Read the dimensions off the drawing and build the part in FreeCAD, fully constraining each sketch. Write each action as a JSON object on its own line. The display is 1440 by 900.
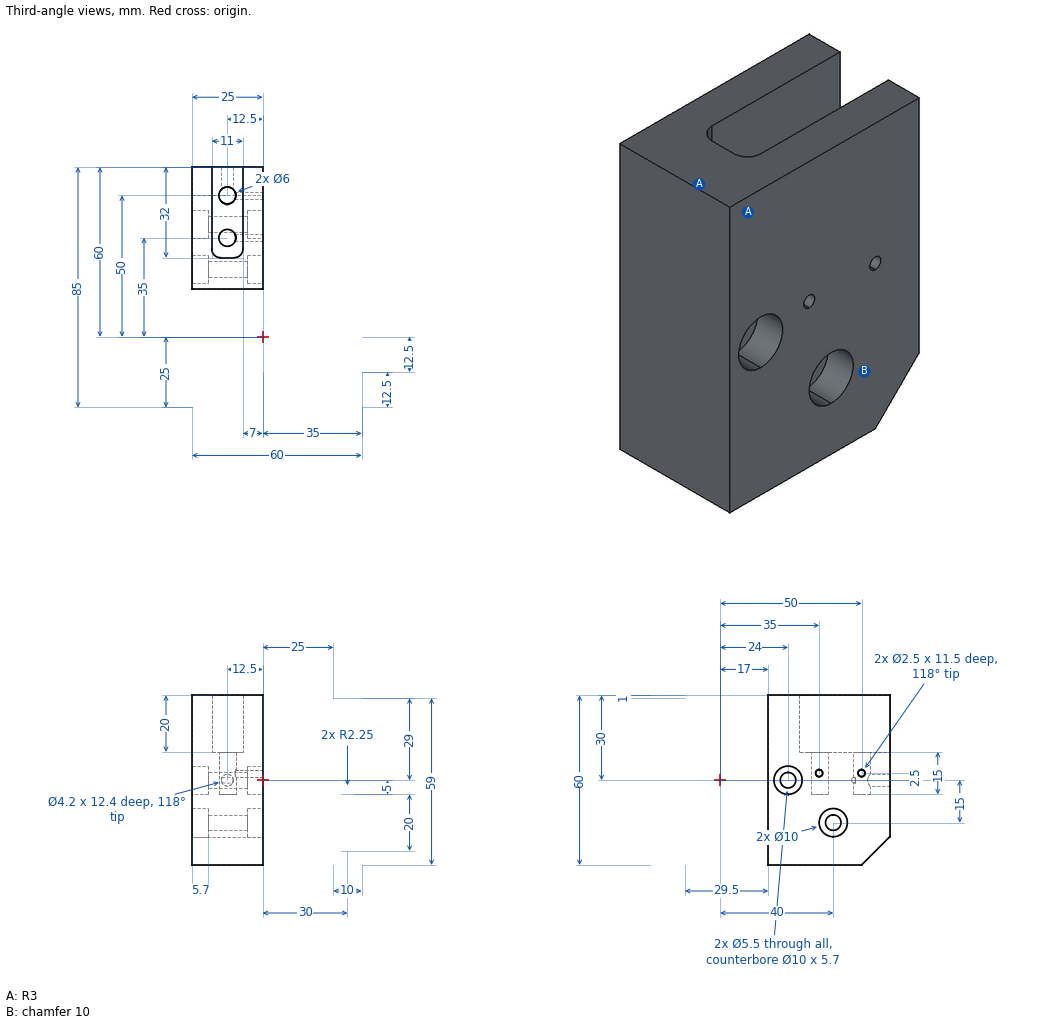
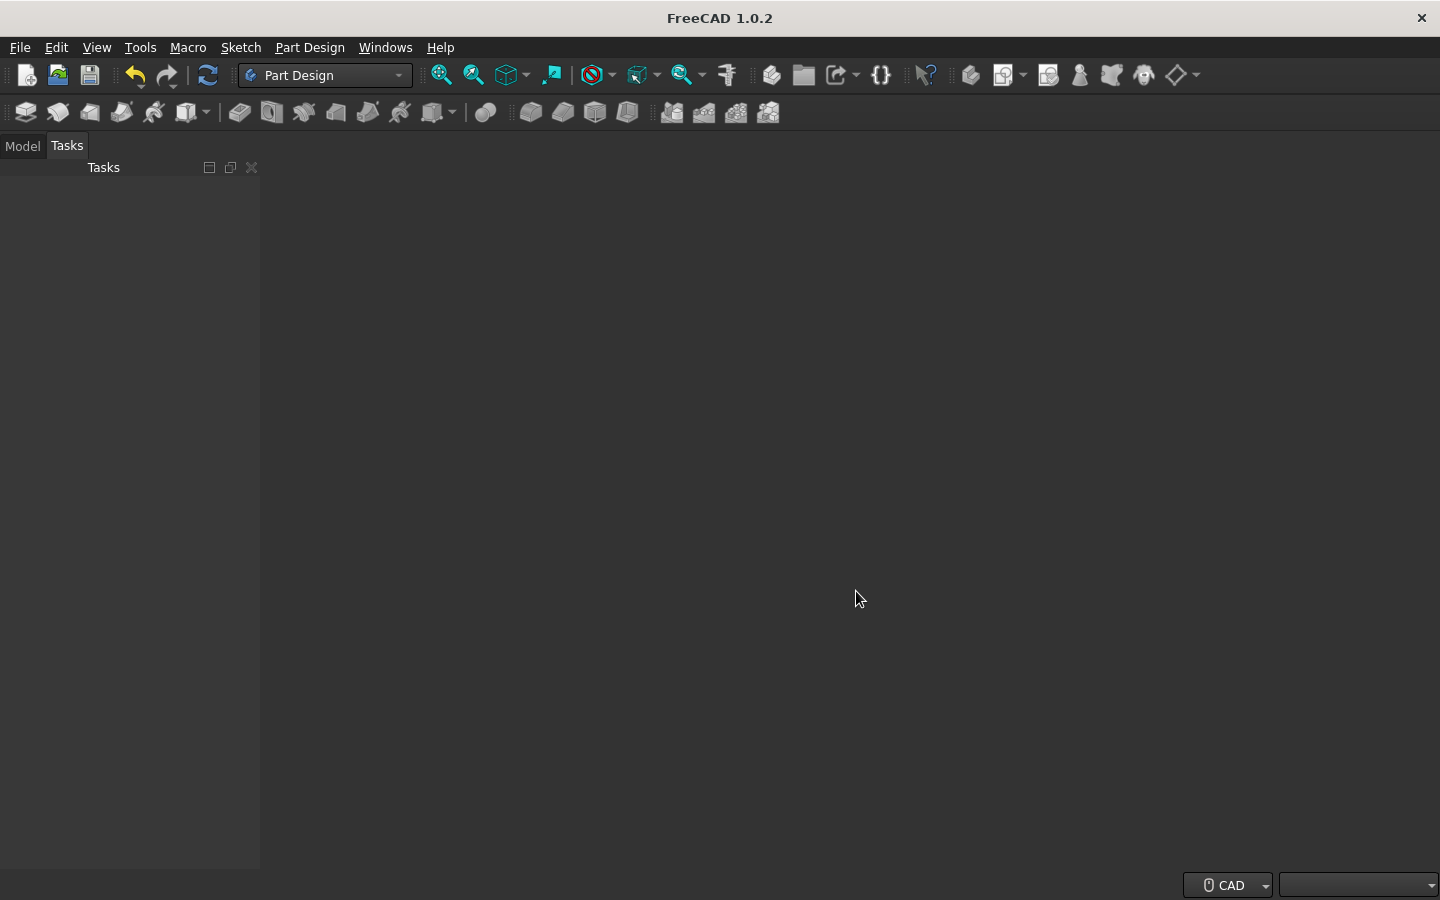
{"action": "left_click", "coordinate": [26, 76]}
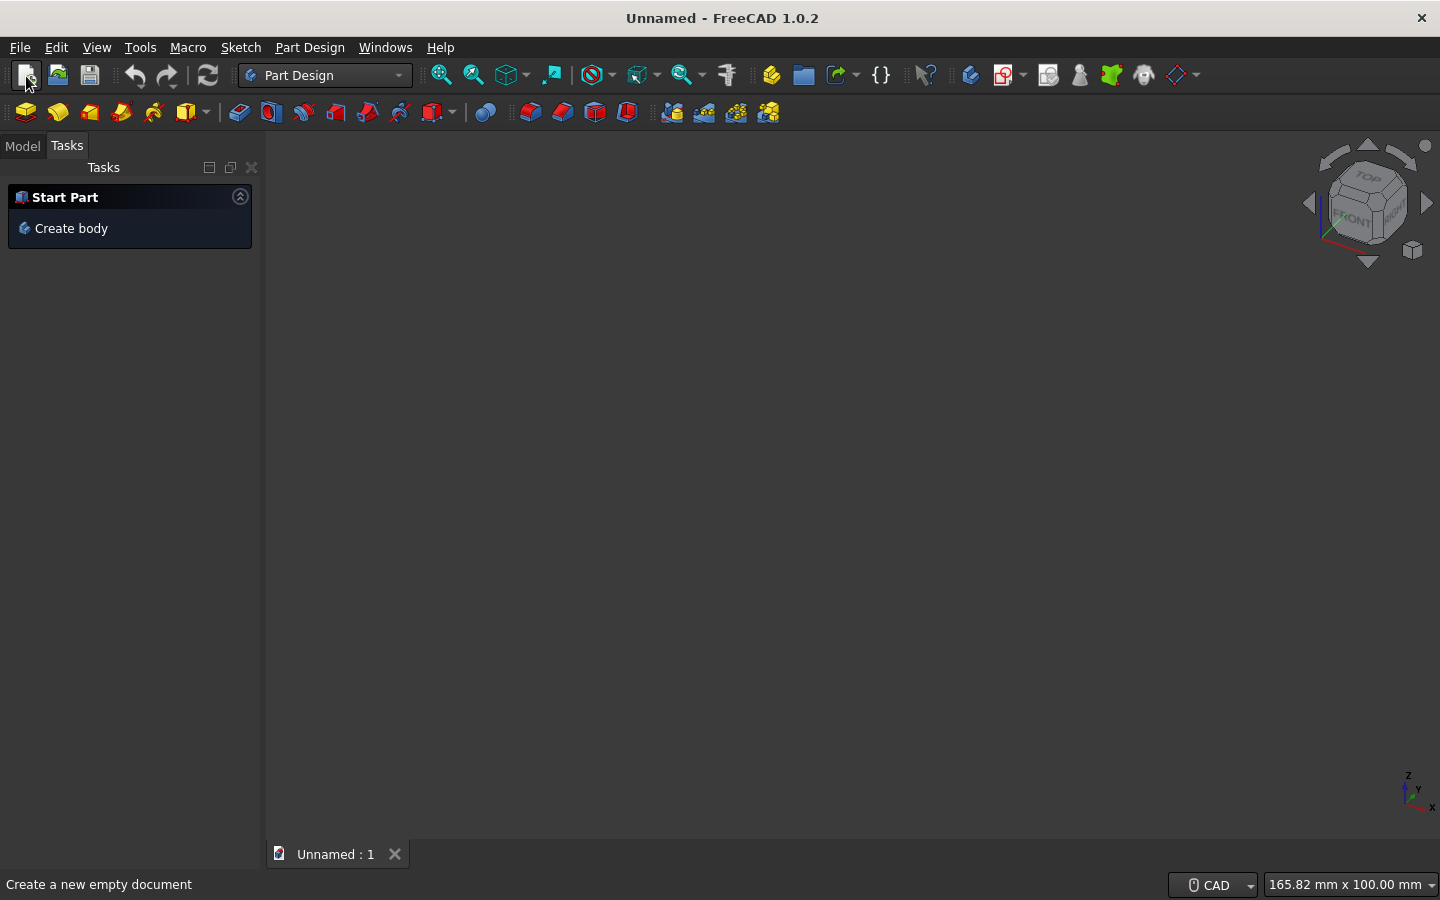
{"action": "left_click", "coordinate": [1004, 76]}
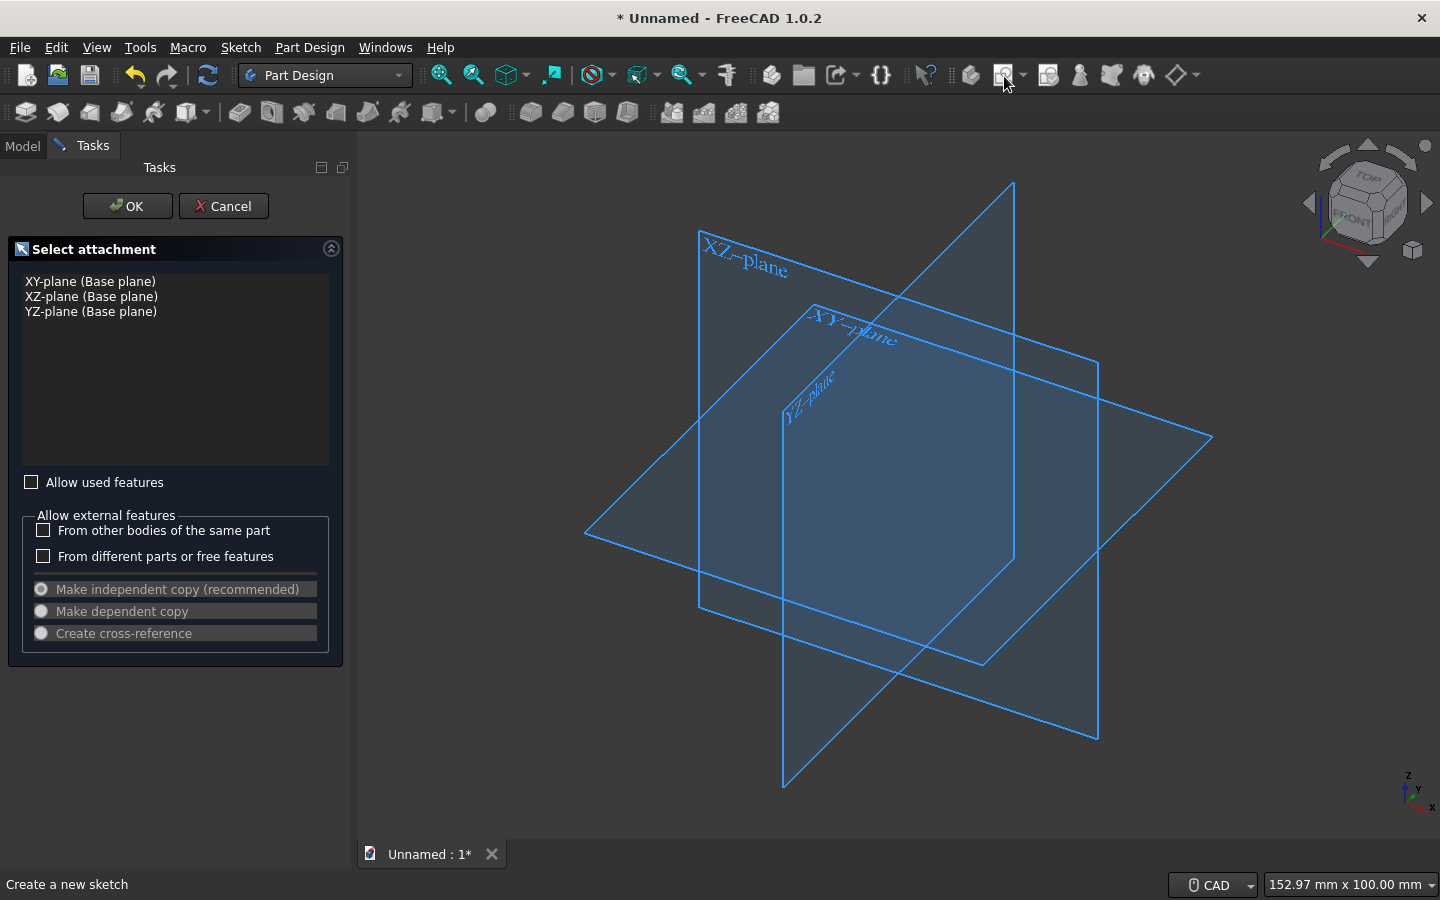
{"action": "left_click", "coordinate": [82, 282]}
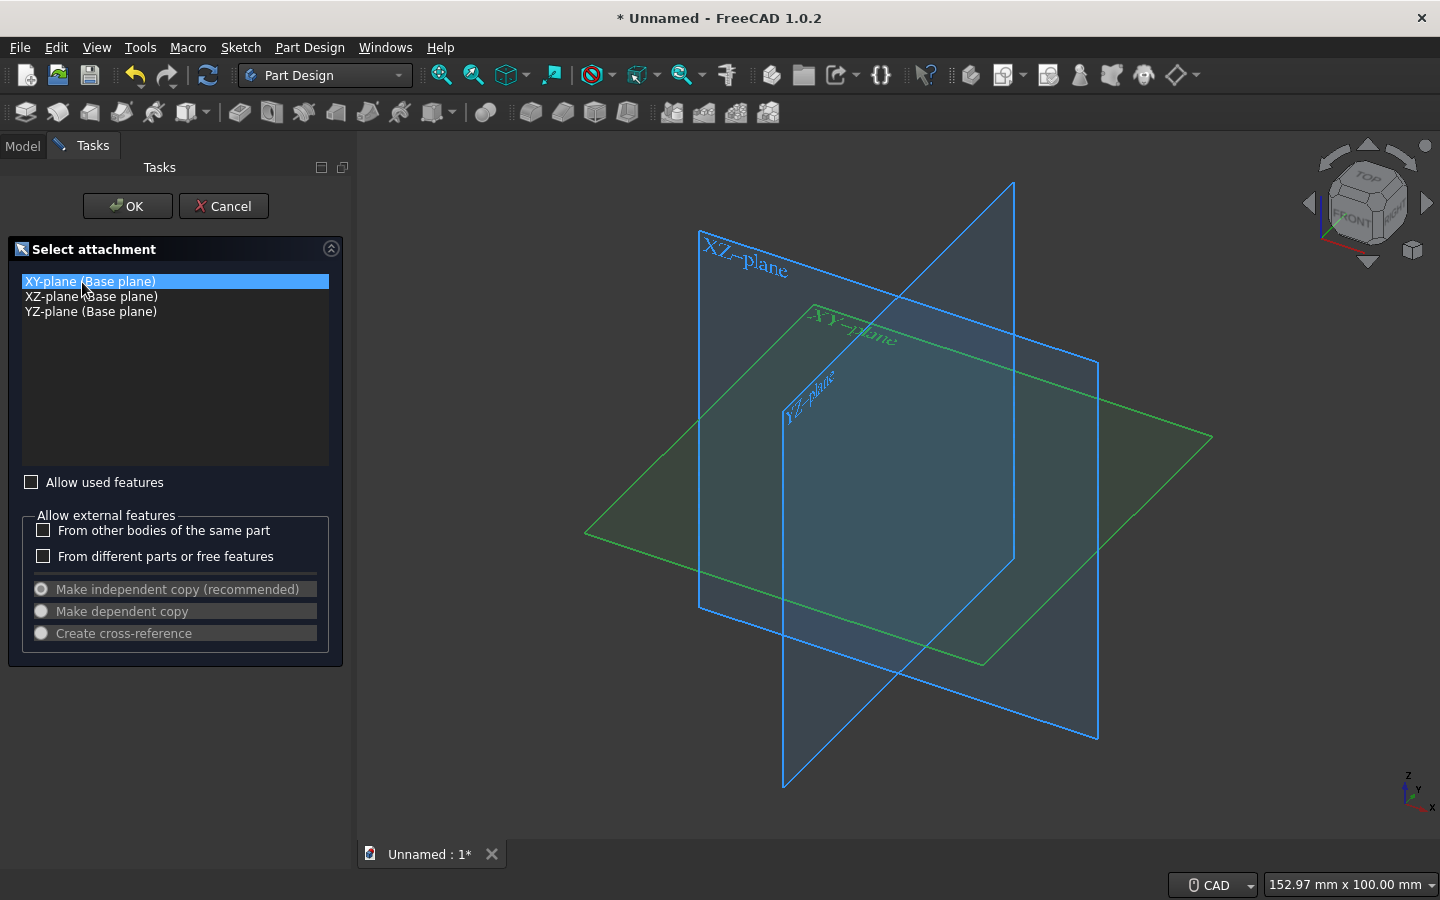
{"action": "left_click", "coordinate": [128, 206]}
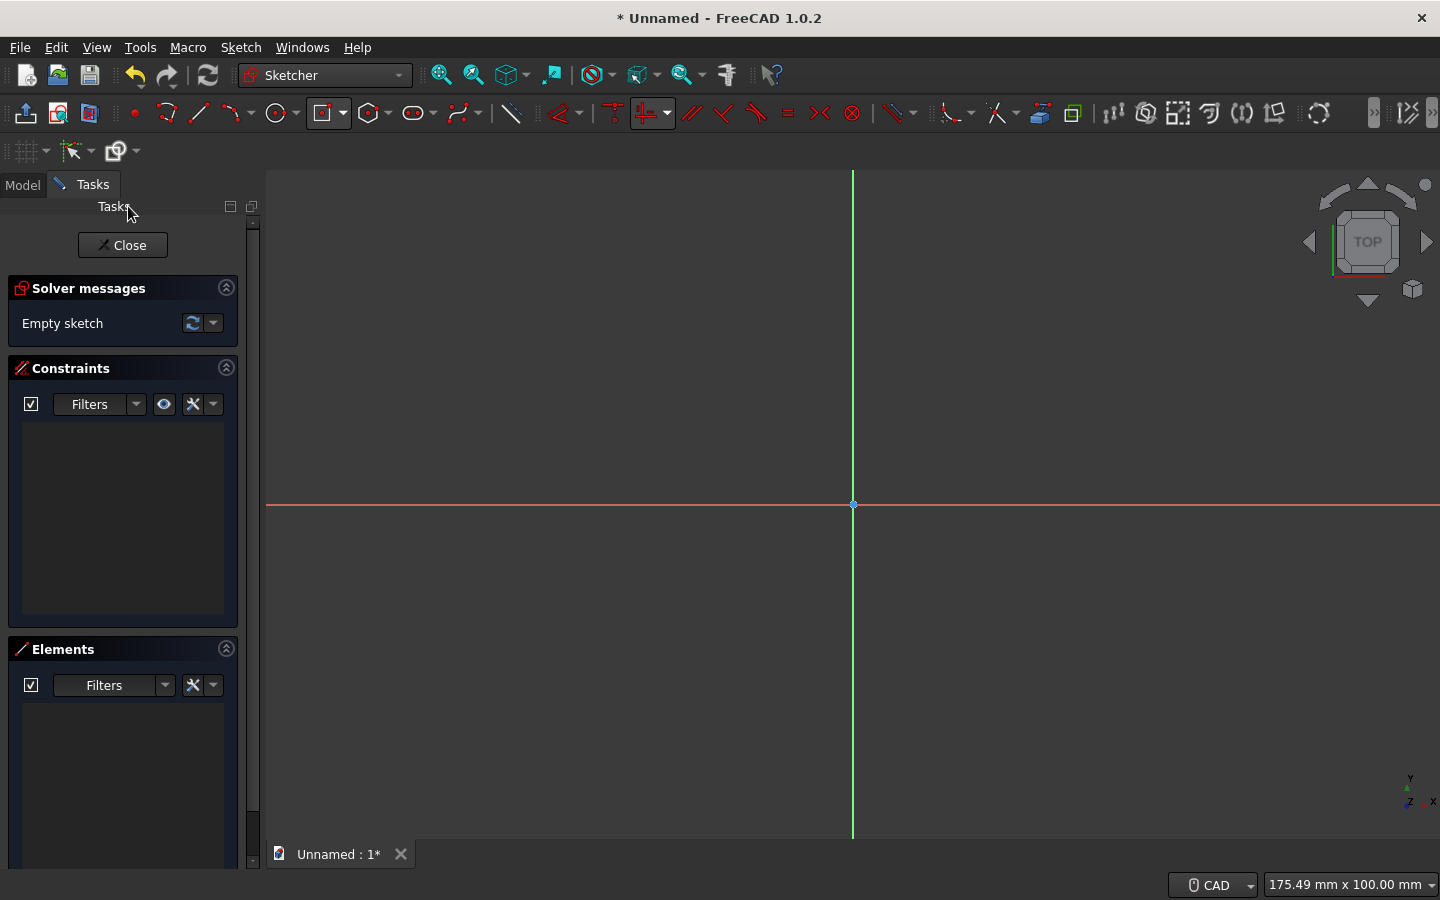
{"action": "scroll", "coordinate": [324, 811], "scroll_direction": "down", "scroll_amount": 1}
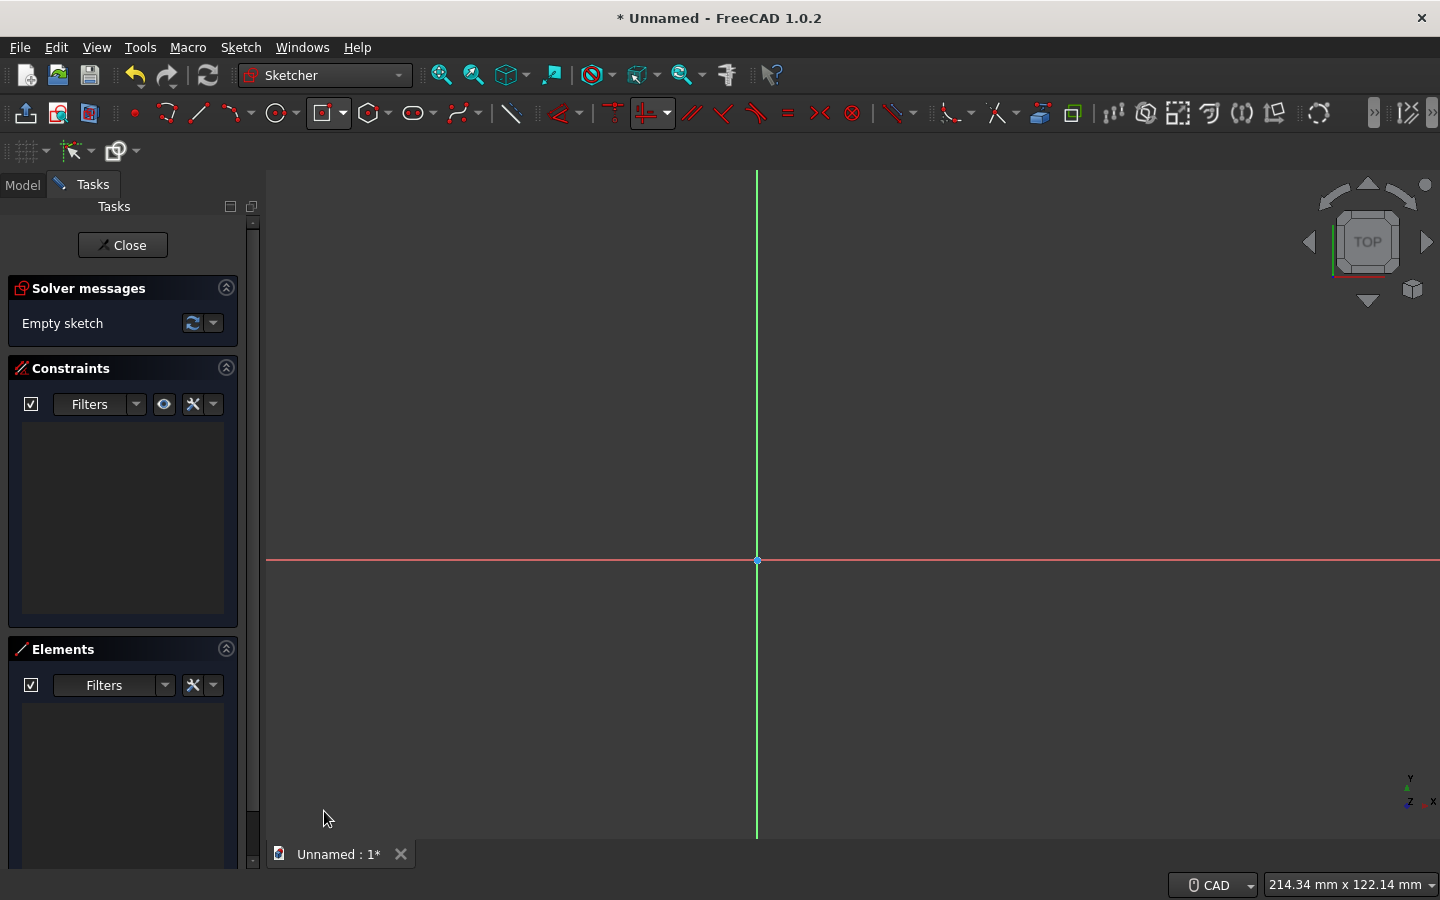
{"action": "left_click", "coordinate": [168, 114]}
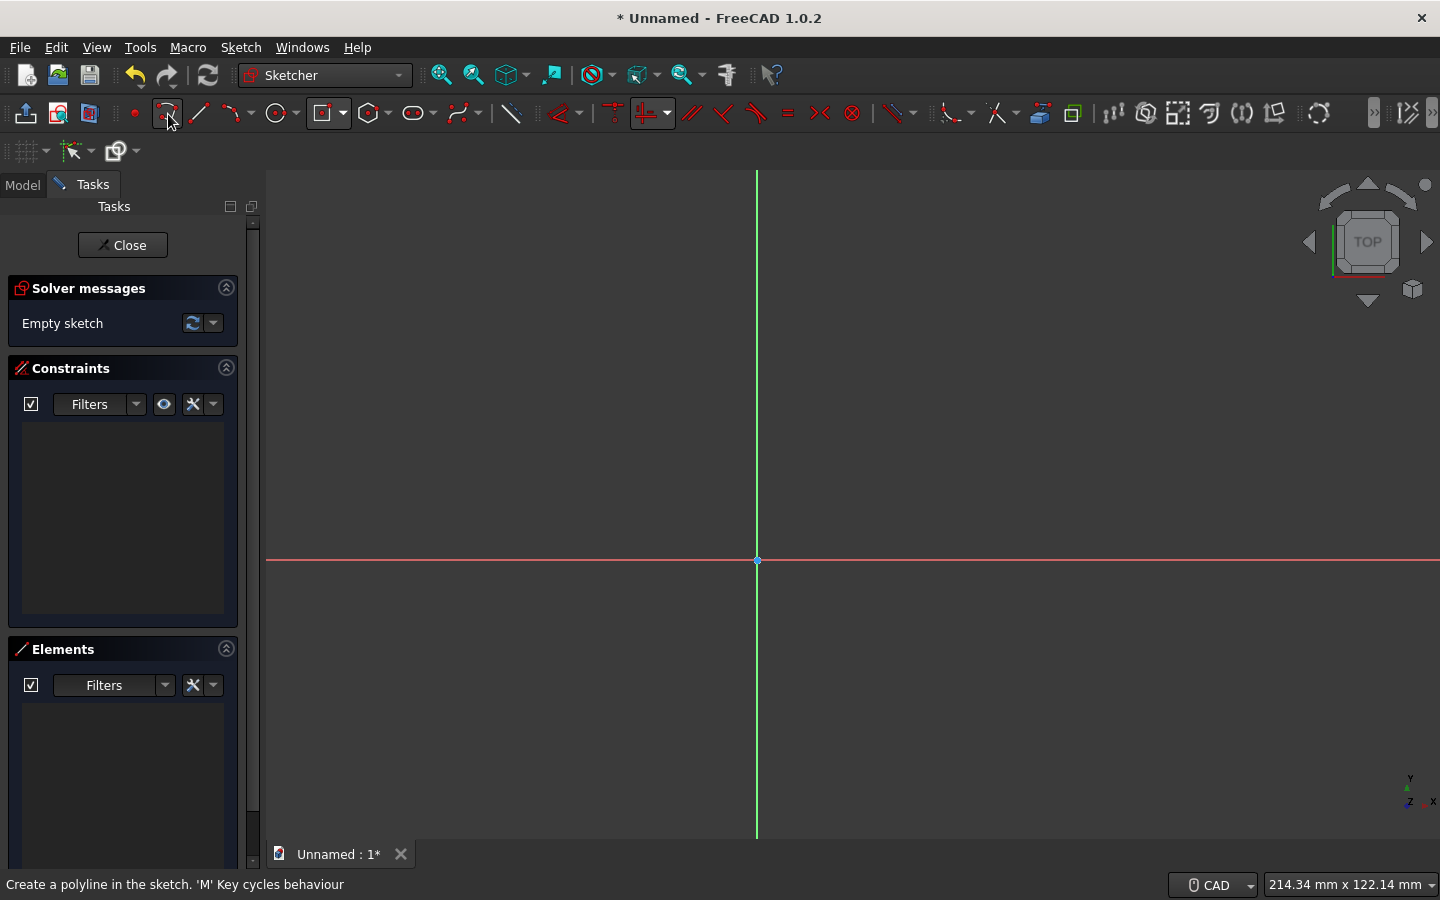
{"action": "left_click", "coordinate": [757, 560]}
{"action": "left_click", "coordinate": [766, 232]}
{"action": "left_click", "coordinate": [620, 232]}
{"action": "left_click", "coordinate": [620, 697]}
{"action": "left_click", "coordinate": [949, 697]}
{"action": "left_click", "coordinate": [949, 551]}
{"action": "left_click", "coordinate": [757, 560]}
{"action": "key", "text": "Escape"}
{"action": "key", "text": "Escape"}